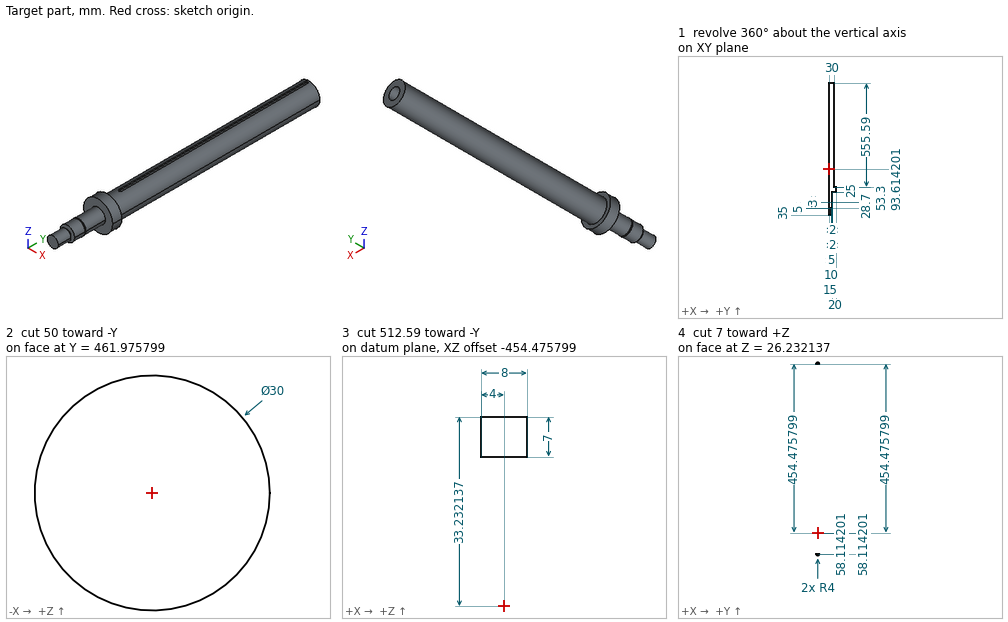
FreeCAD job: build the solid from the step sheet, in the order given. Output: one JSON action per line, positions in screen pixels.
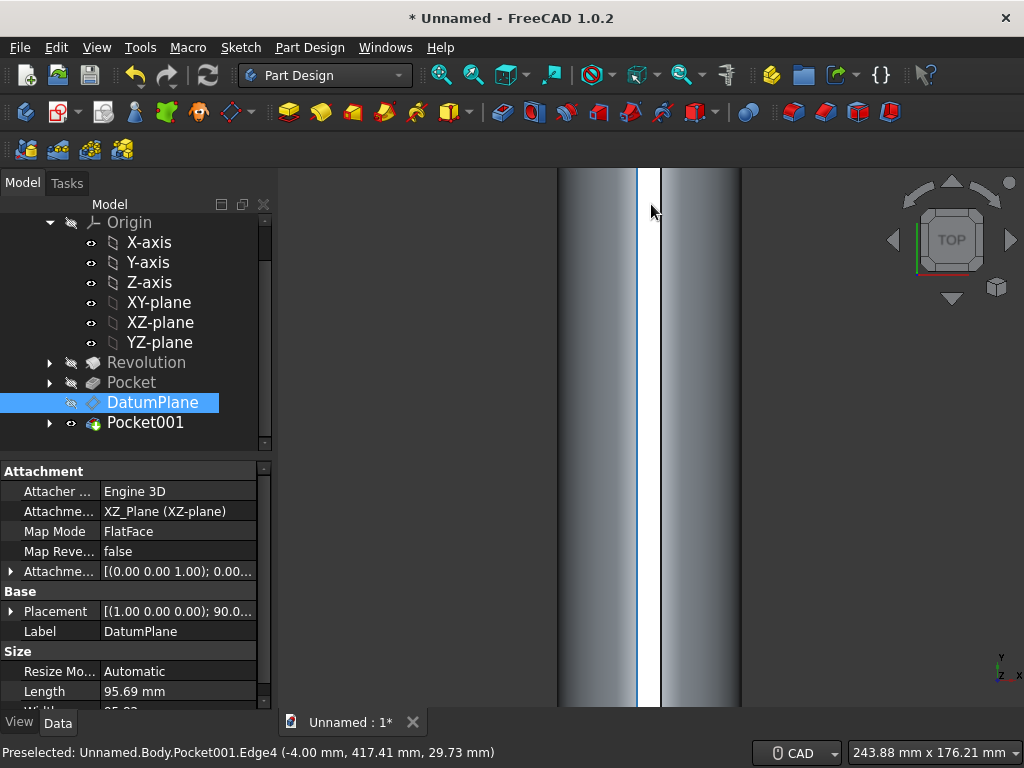
{"action": "left_click", "coordinate": [649, 205]}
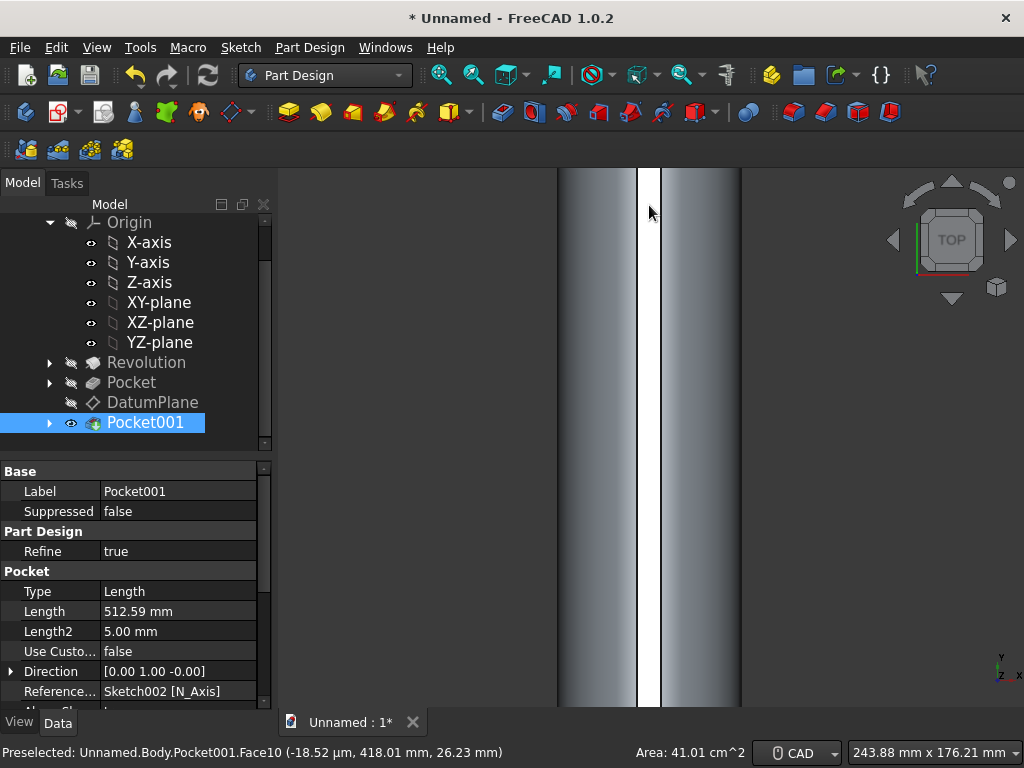
{"action": "left_click", "coordinate": [58, 112]}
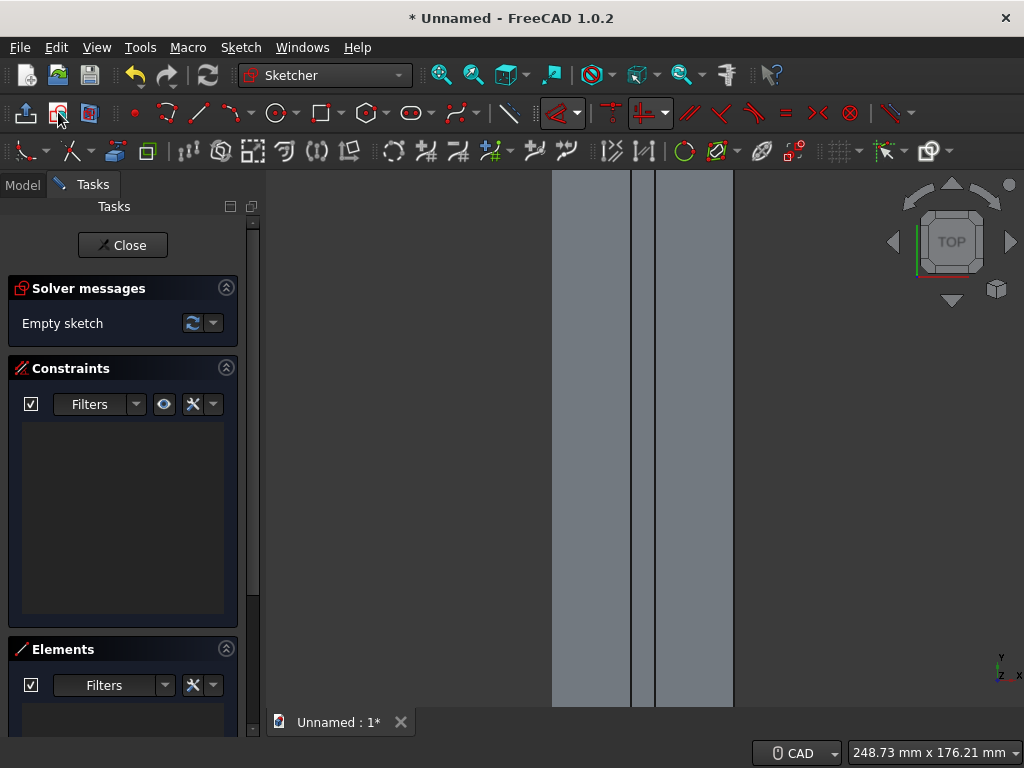
{"action": "scroll", "coordinate": [560, 327], "scroll_direction": "down", "scroll_amount": 8}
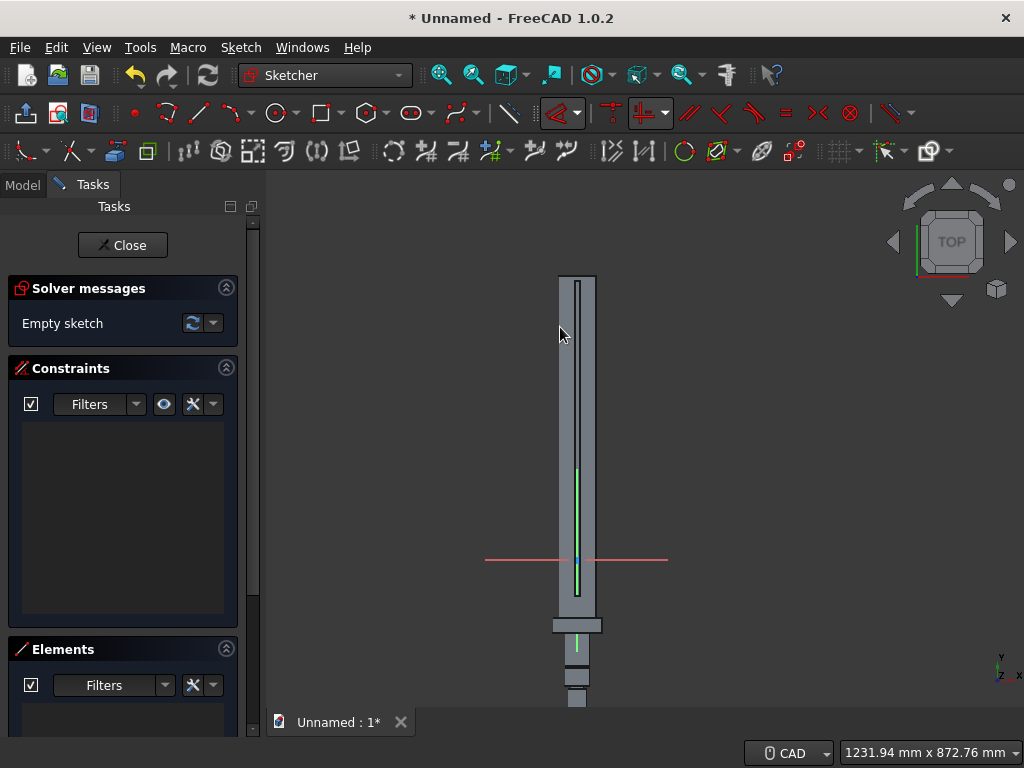
{"action": "key", "text": "g l"}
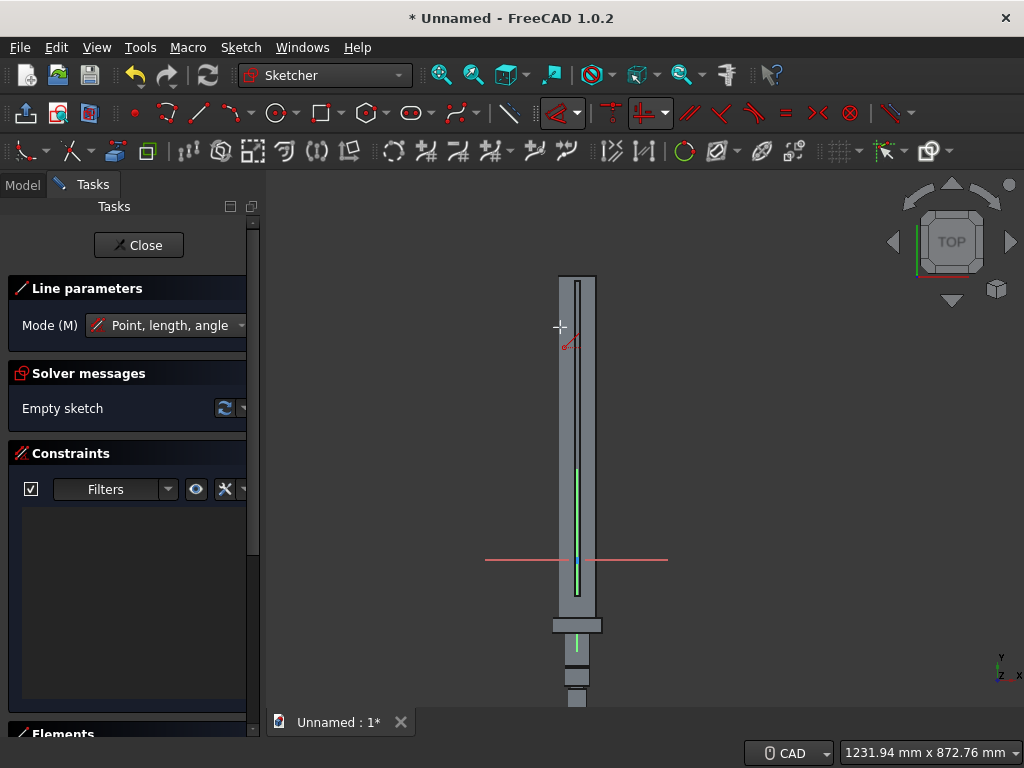
{"action": "scroll", "coordinate": [580, 596], "scroll_direction": "up", "scroll_amount": 10}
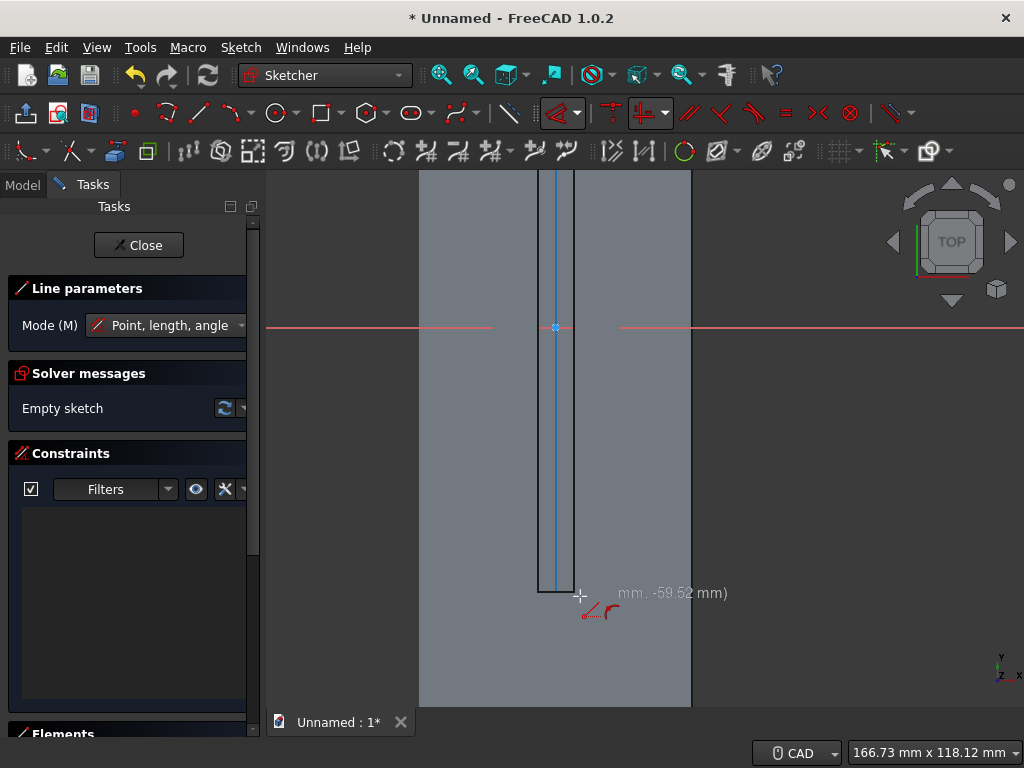
{"action": "left_click", "coordinate": [574, 592]}
{"action": "left_click", "coordinate": [538, 592]}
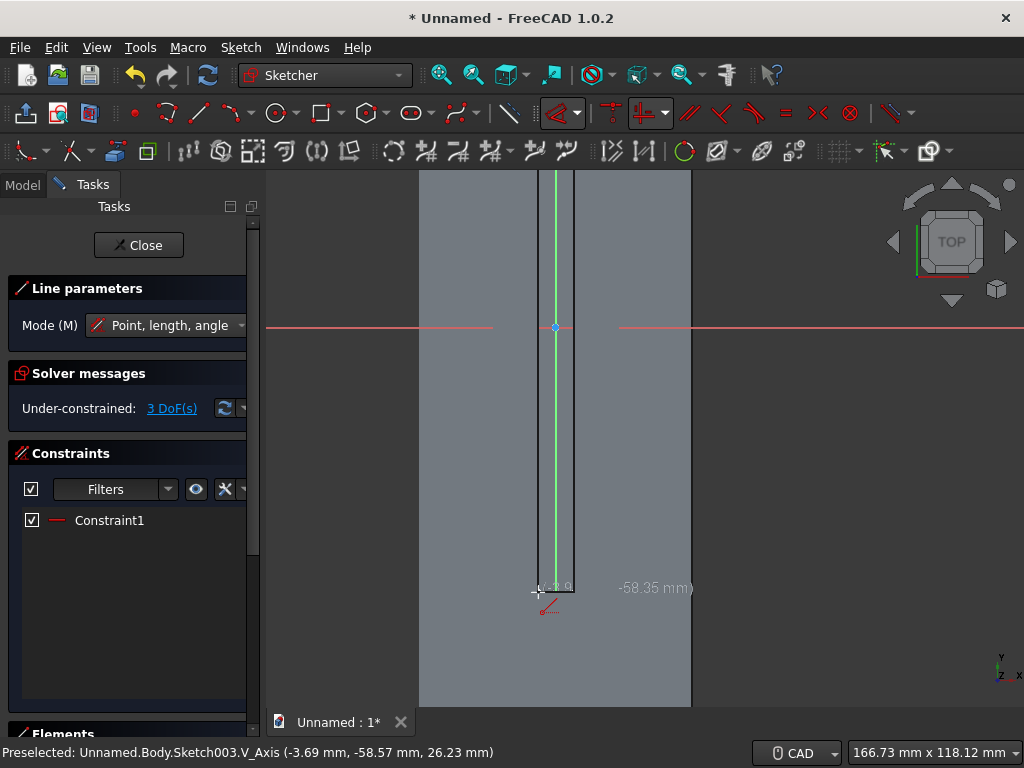
{"action": "key", "text": "g 3 a"}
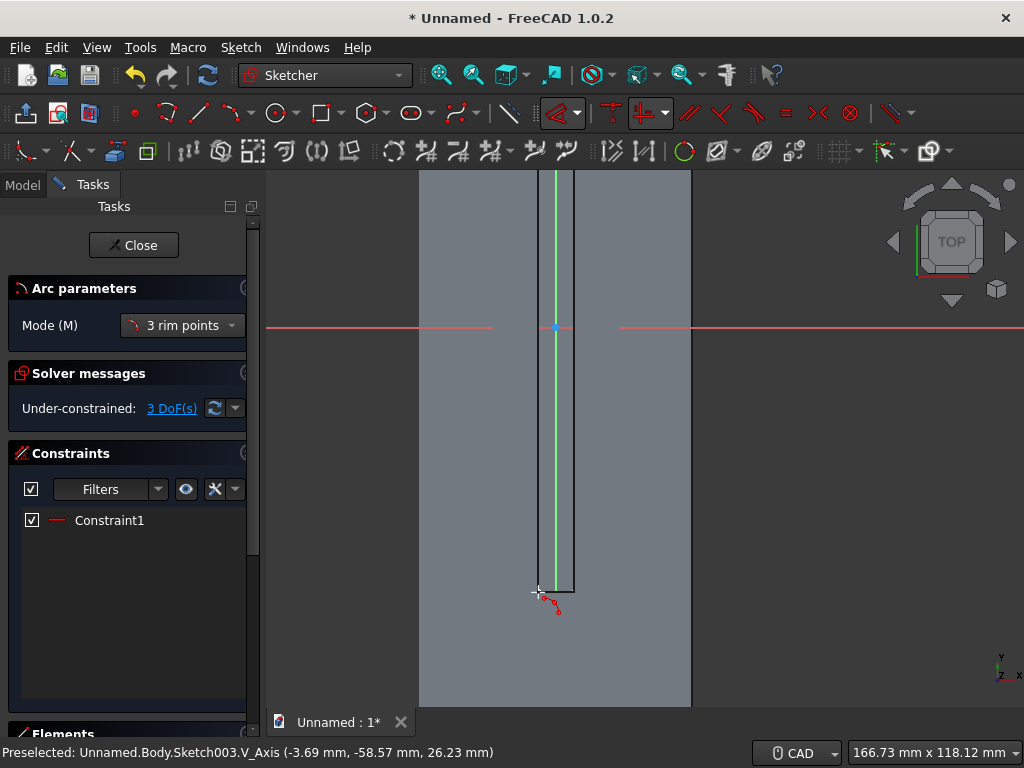
{"action": "left_click", "coordinate": [538, 593]}
{"action": "left_click", "coordinate": [574, 593]}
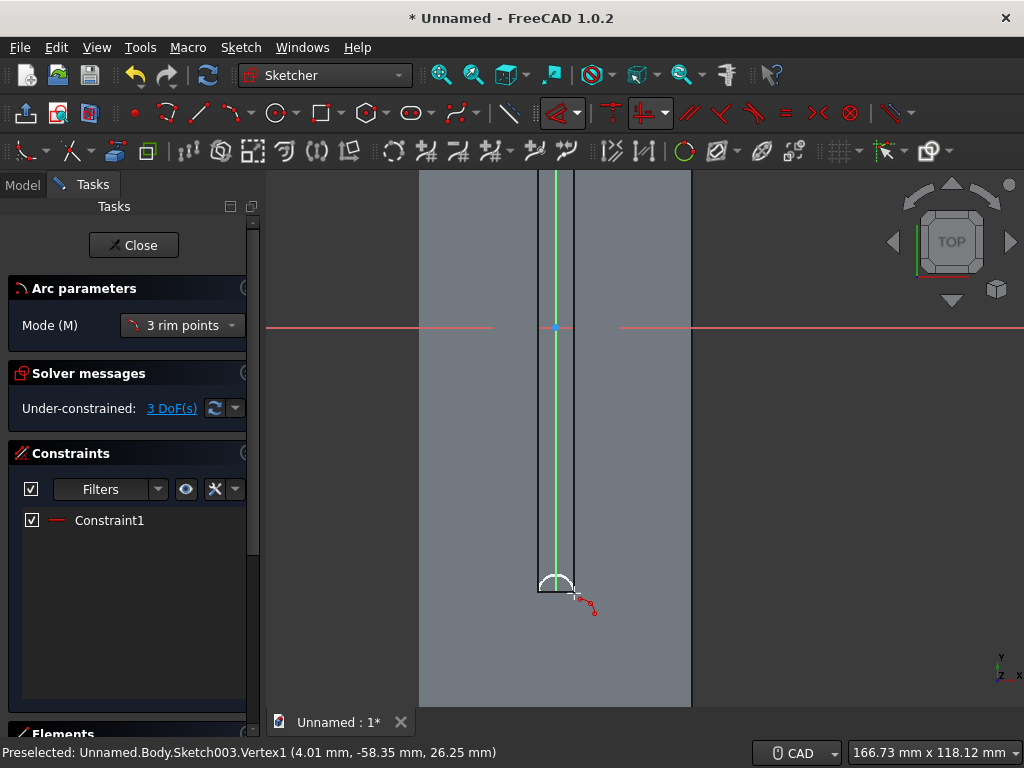
{"action": "scroll", "coordinate": [545, 607], "scroll_direction": "up", "scroll_amount": 2}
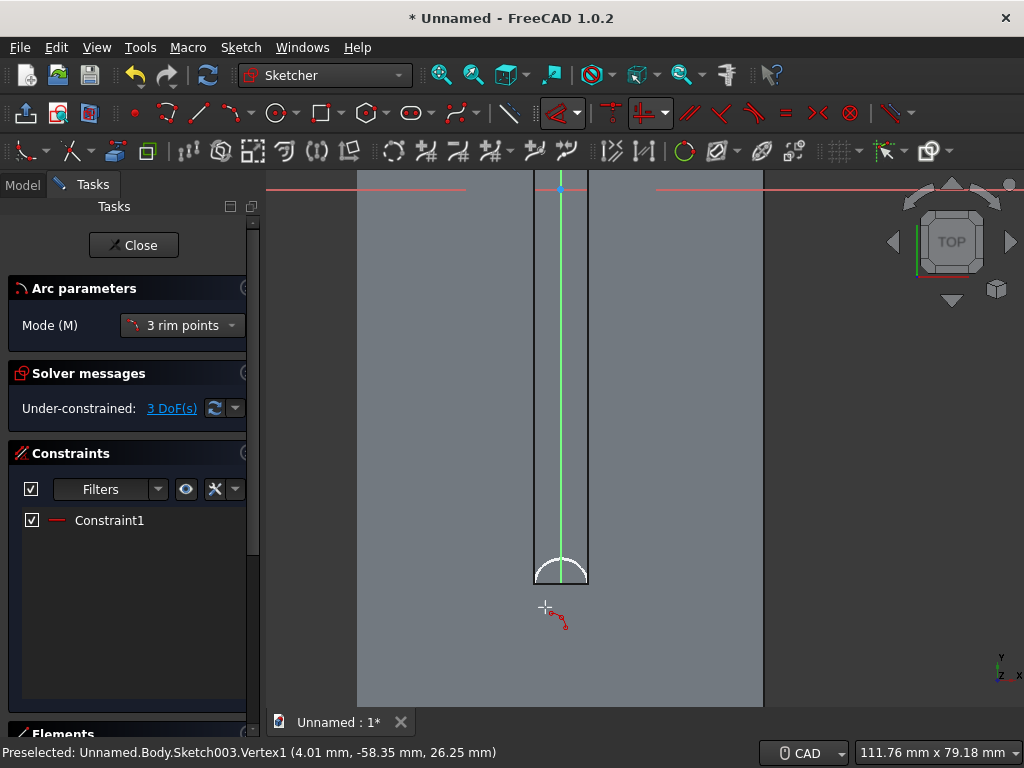
{"action": "left_click", "coordinate": [545, 606]}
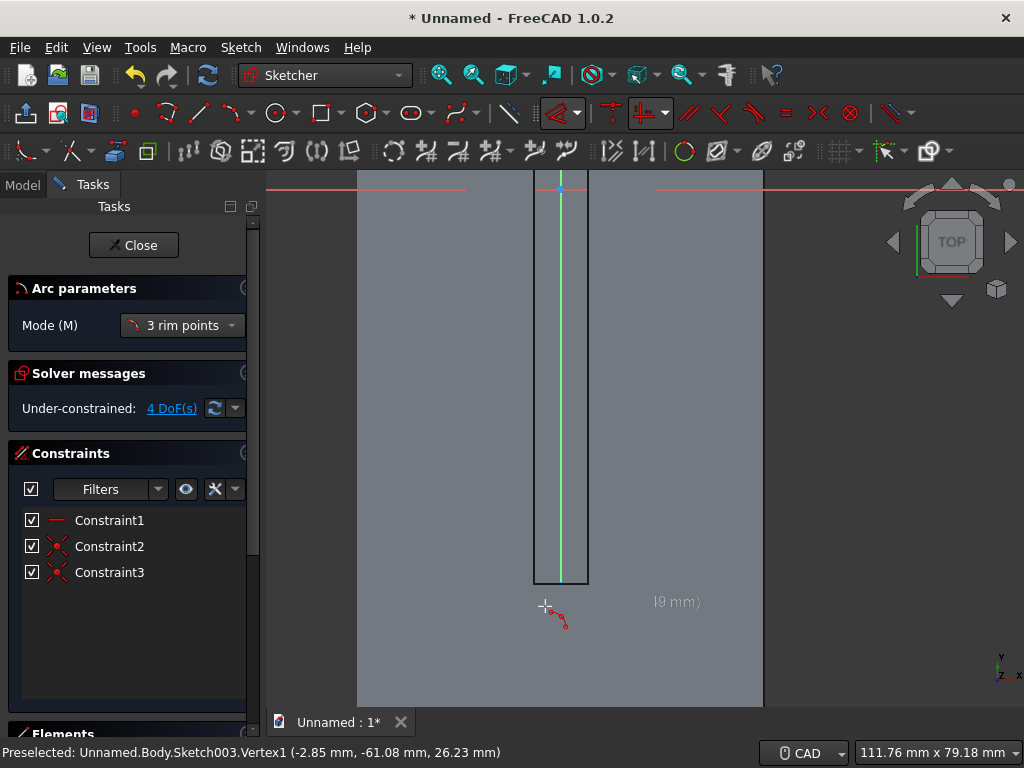
{"action": "key", "text": "g l"}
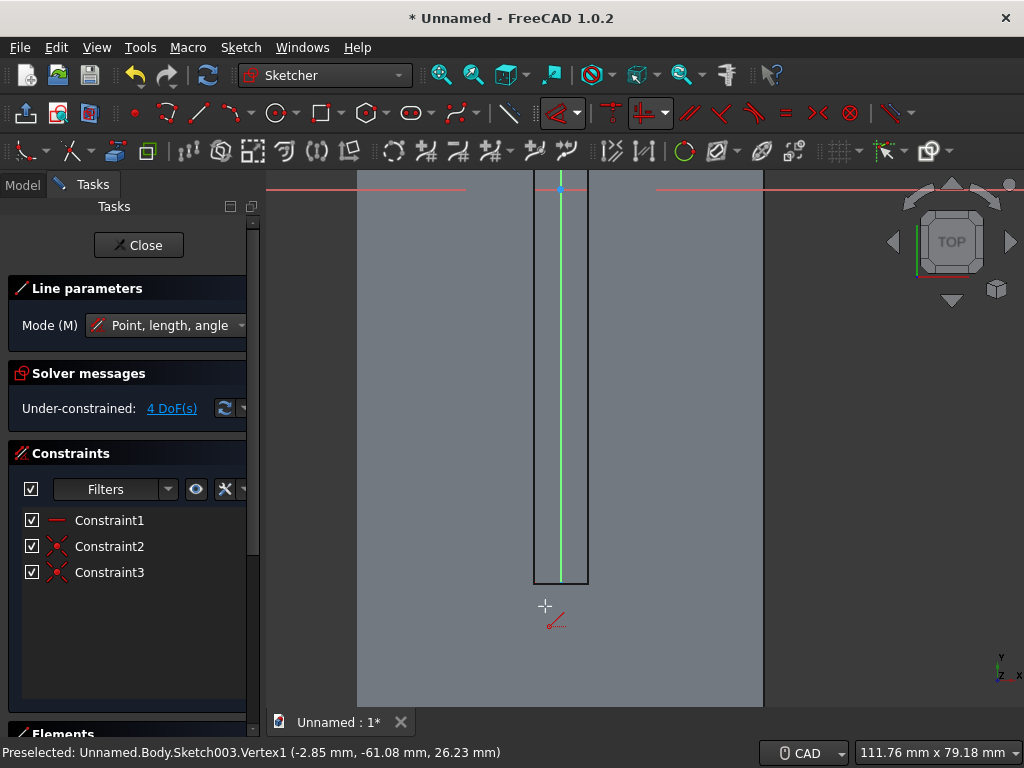
{"action": "scroll", "coordinate": [578, 597], "scroll_direction": "down", "scroll_amount": 12}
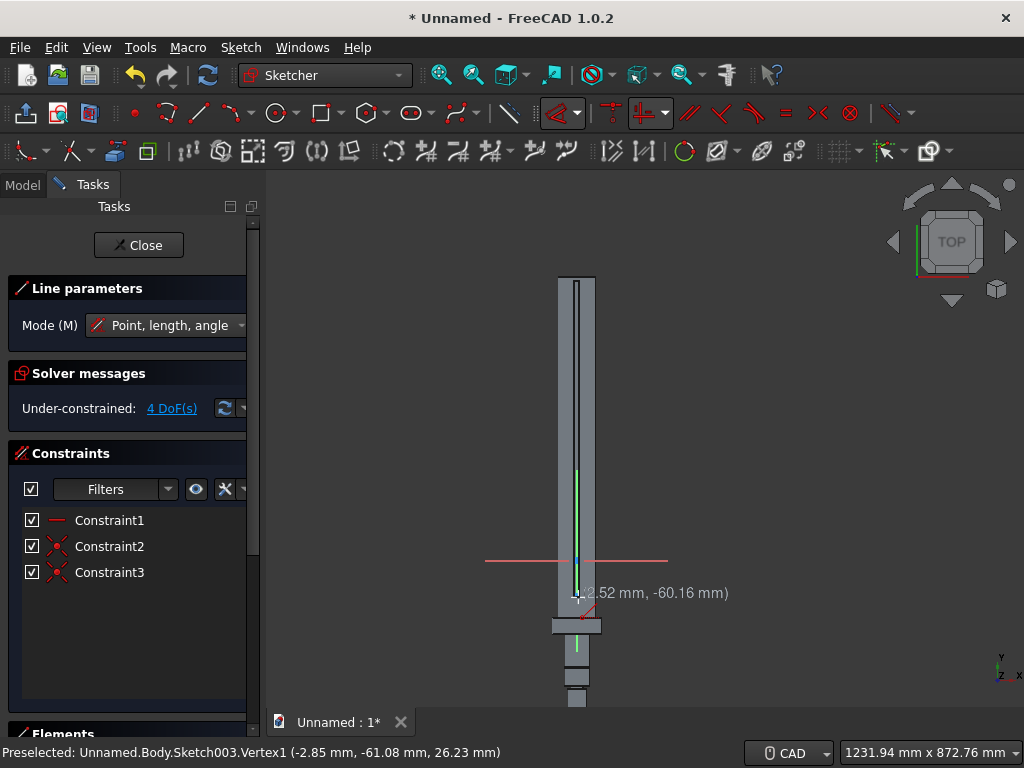
{"action": "scroll", "coordinate": [574, 281], "scroll_direction": "up", "scroll_amount": 10}